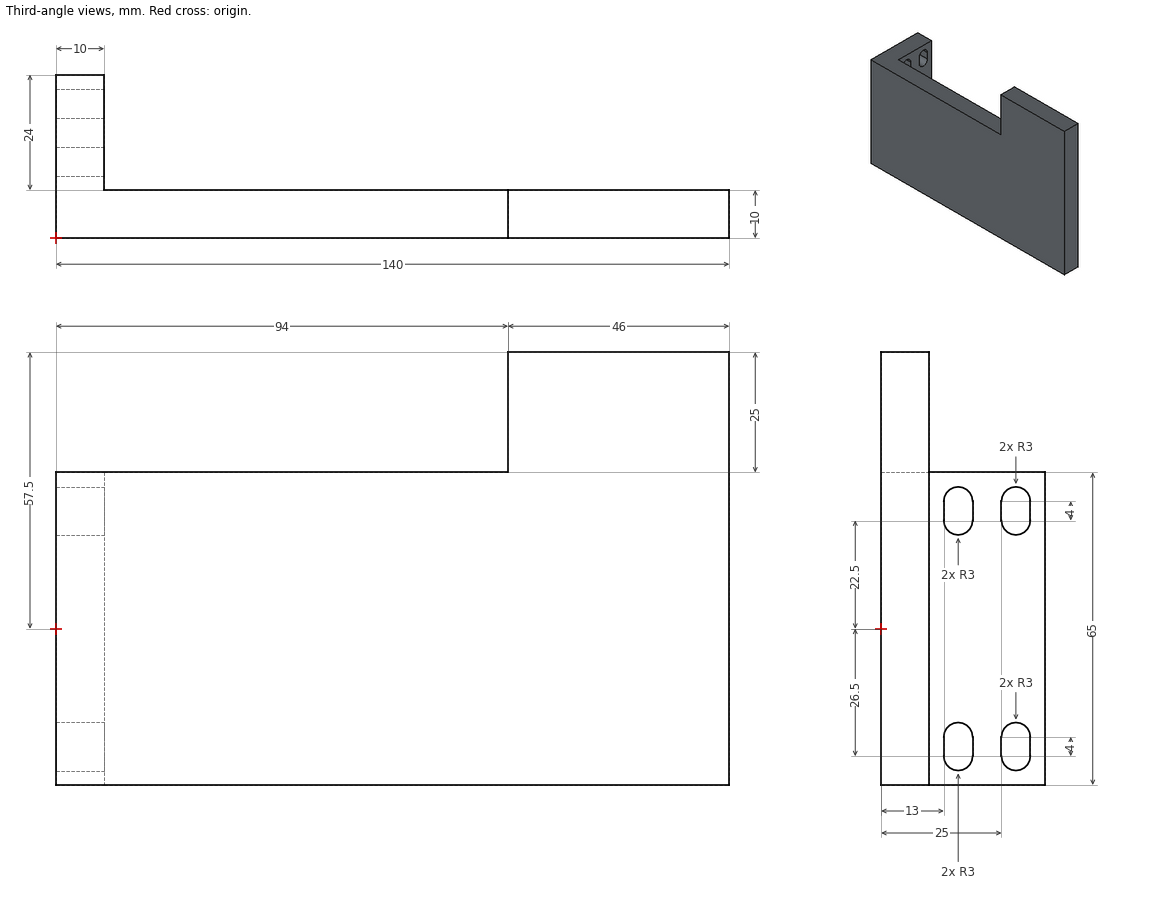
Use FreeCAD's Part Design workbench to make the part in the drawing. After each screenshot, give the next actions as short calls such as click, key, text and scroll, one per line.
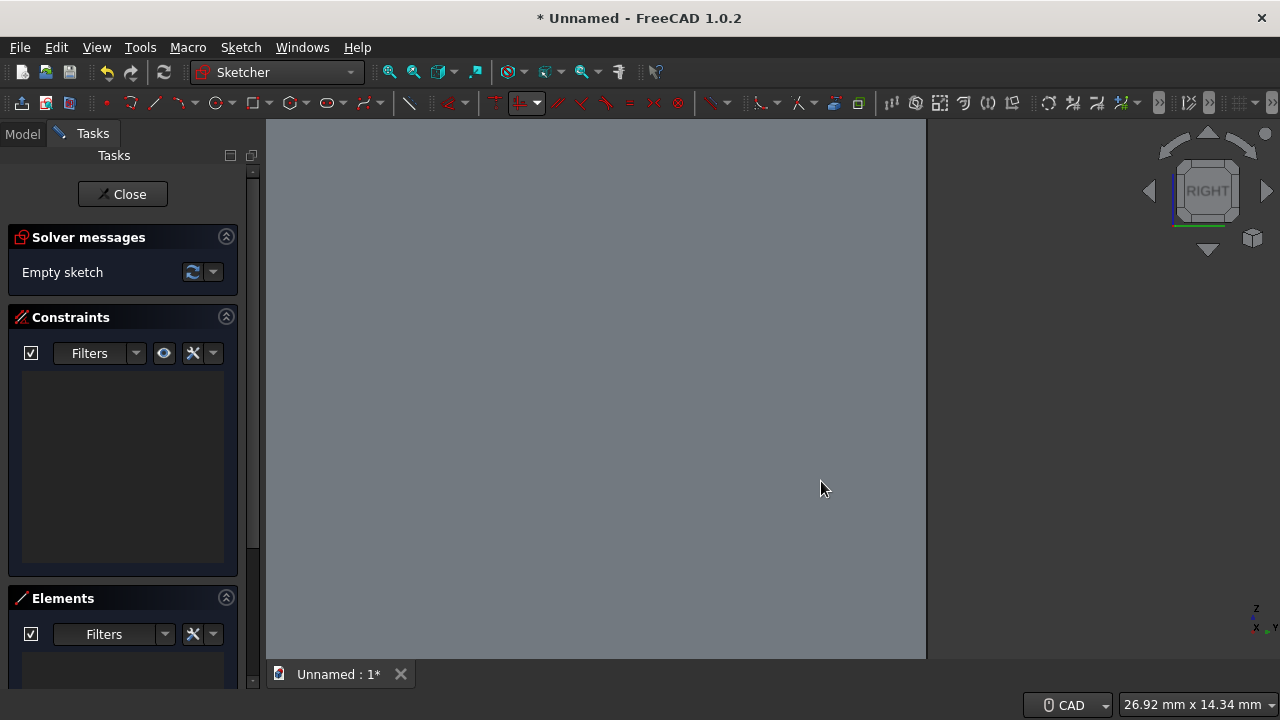
key(g)
key(s)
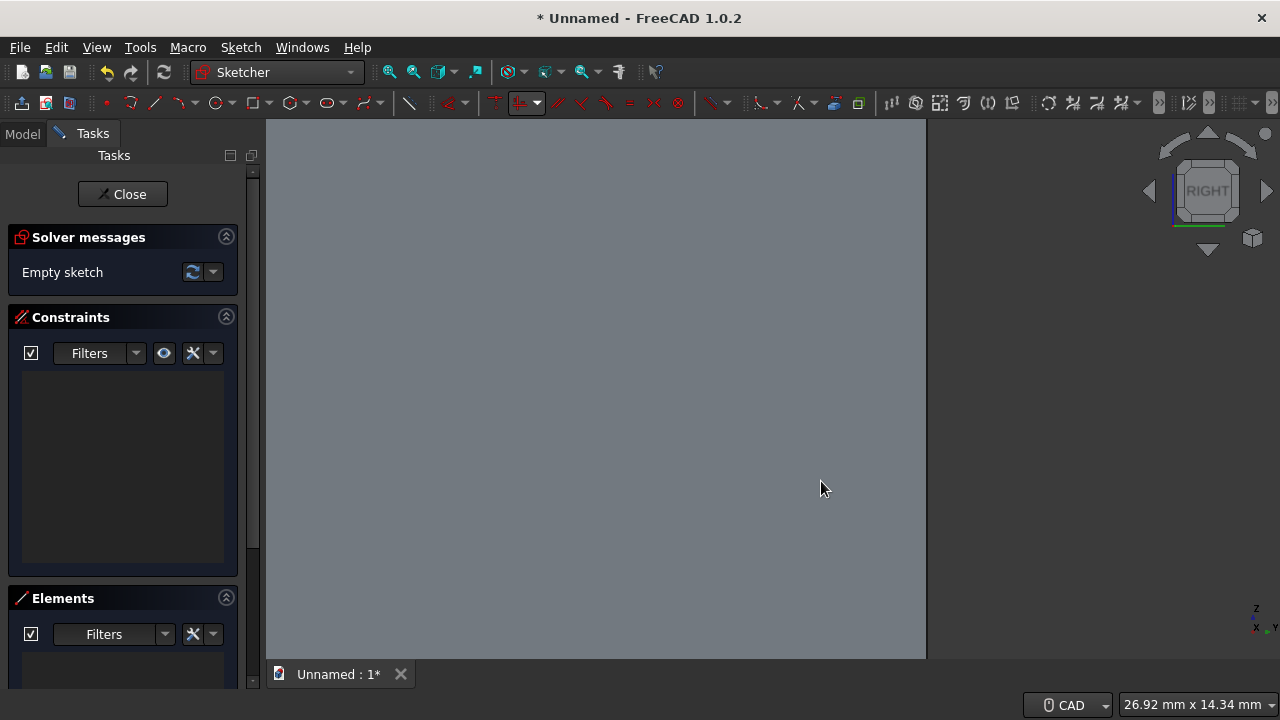
click(701, 458)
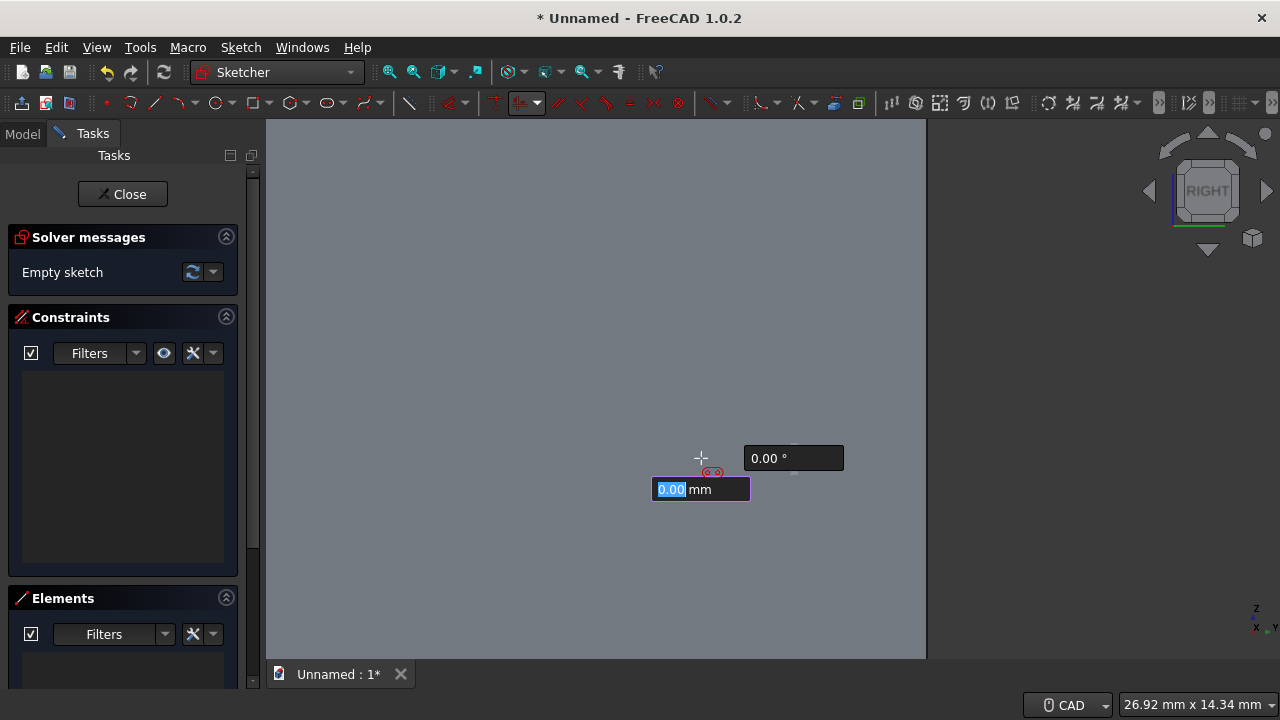
click(701, 308)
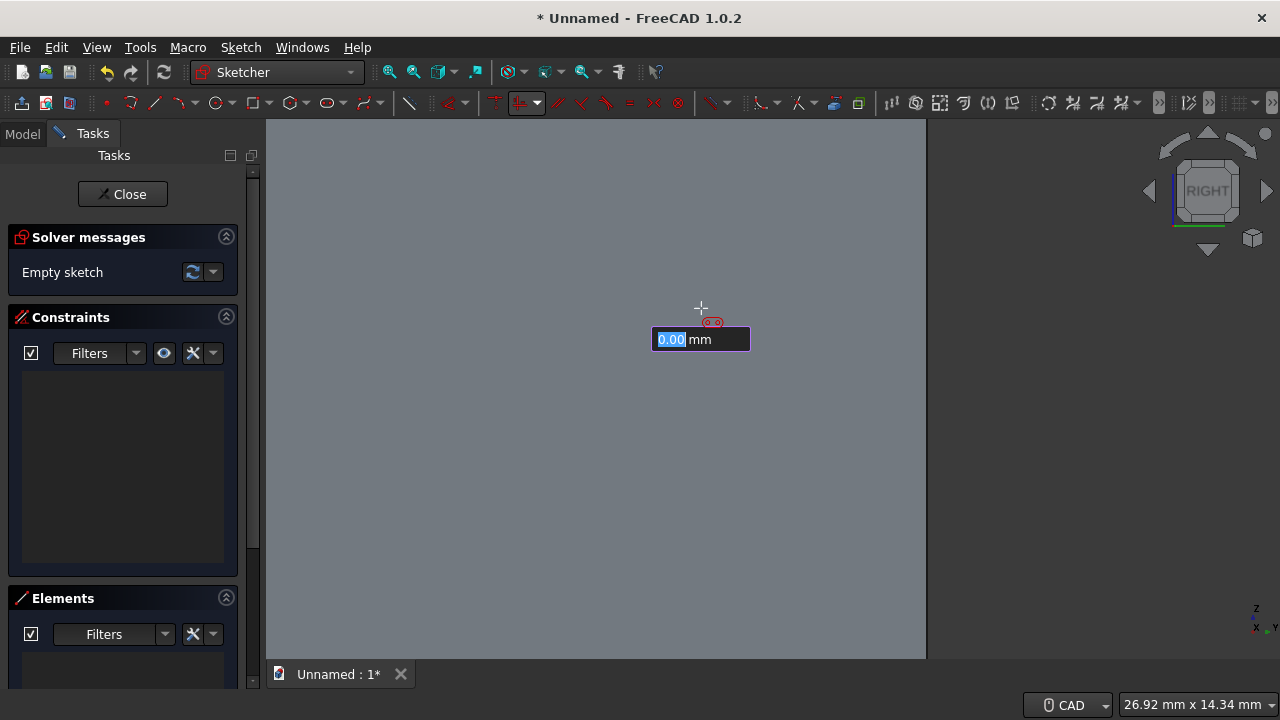
click(814, 383)
key(Escape)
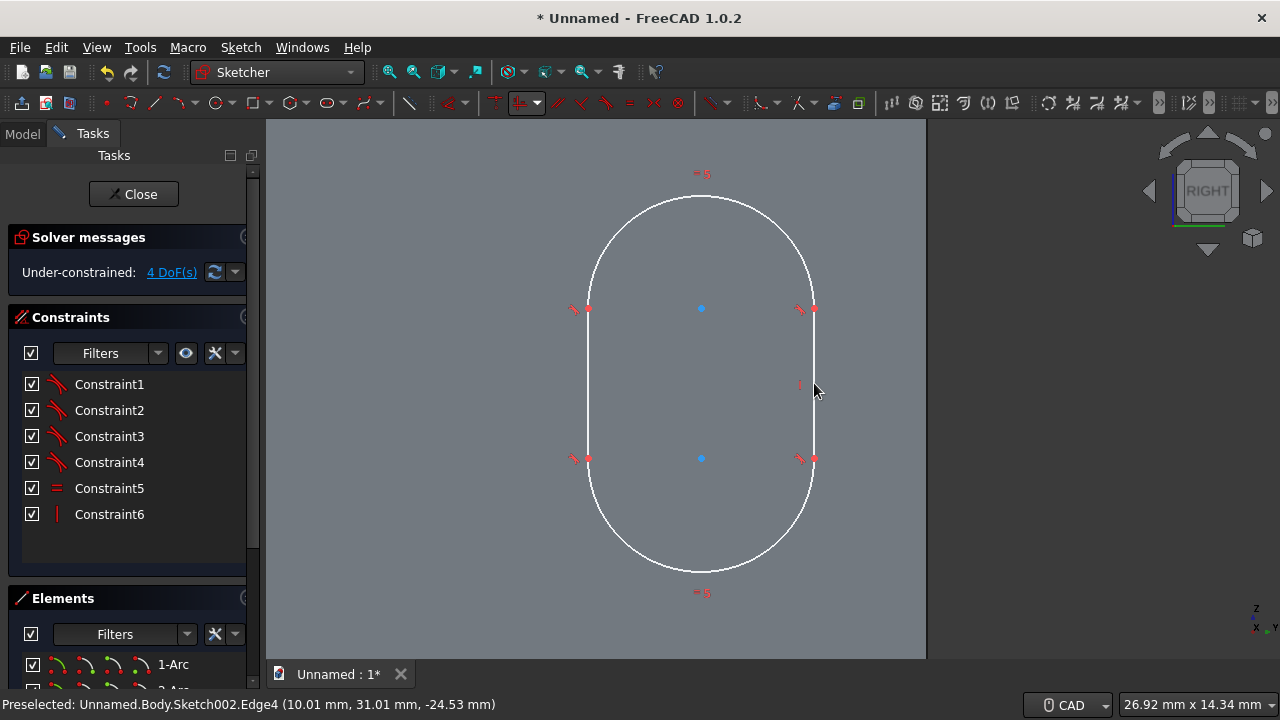
click(448, 104)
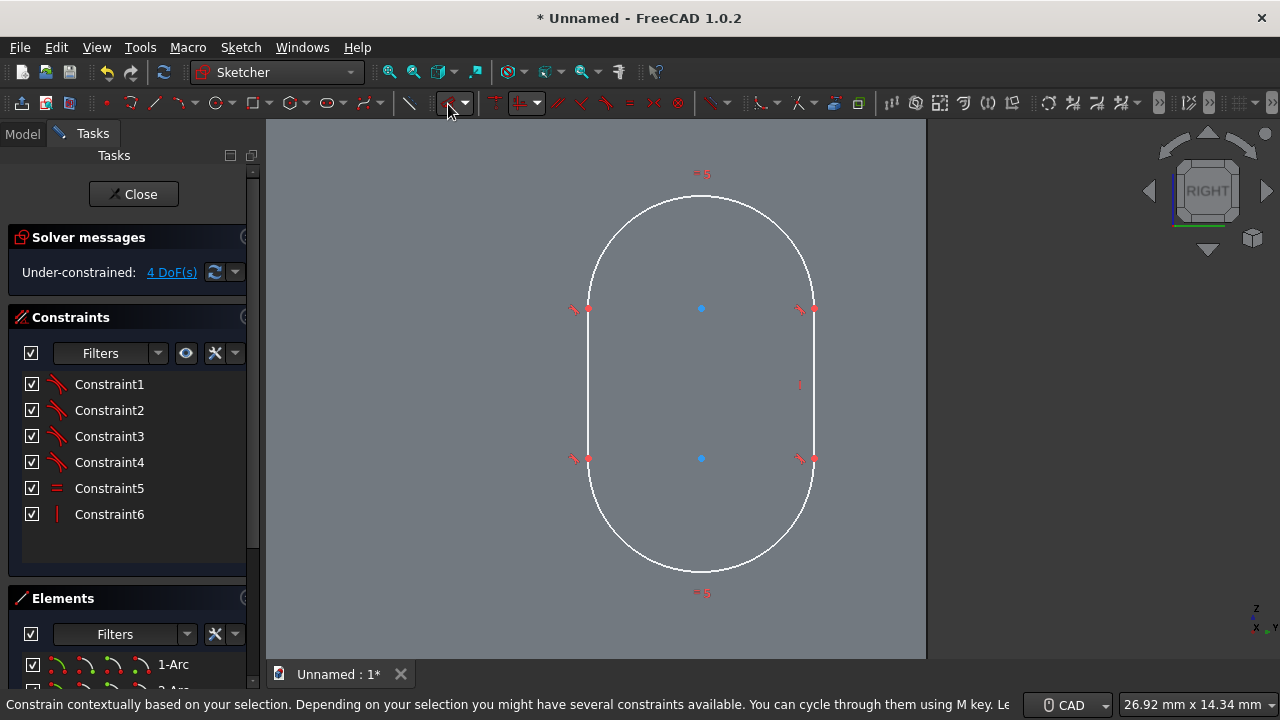
click(635, 550)
click(616, 576)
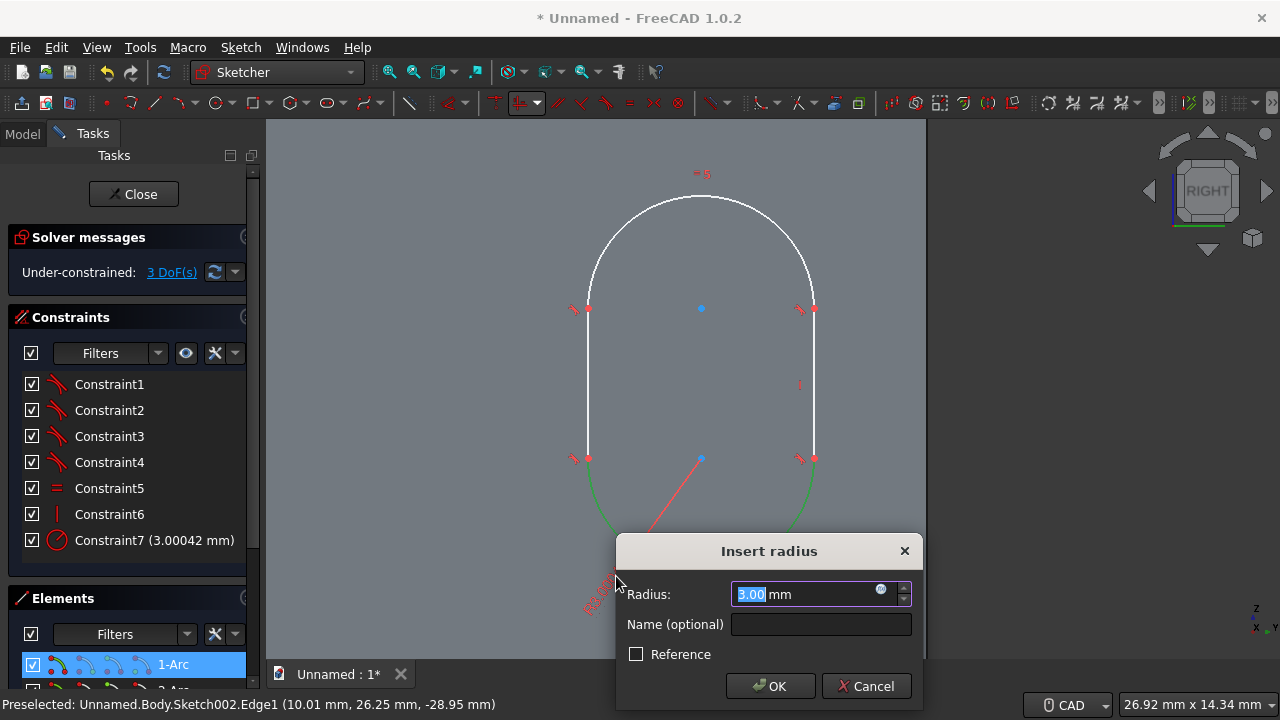
text(3)
key(Return)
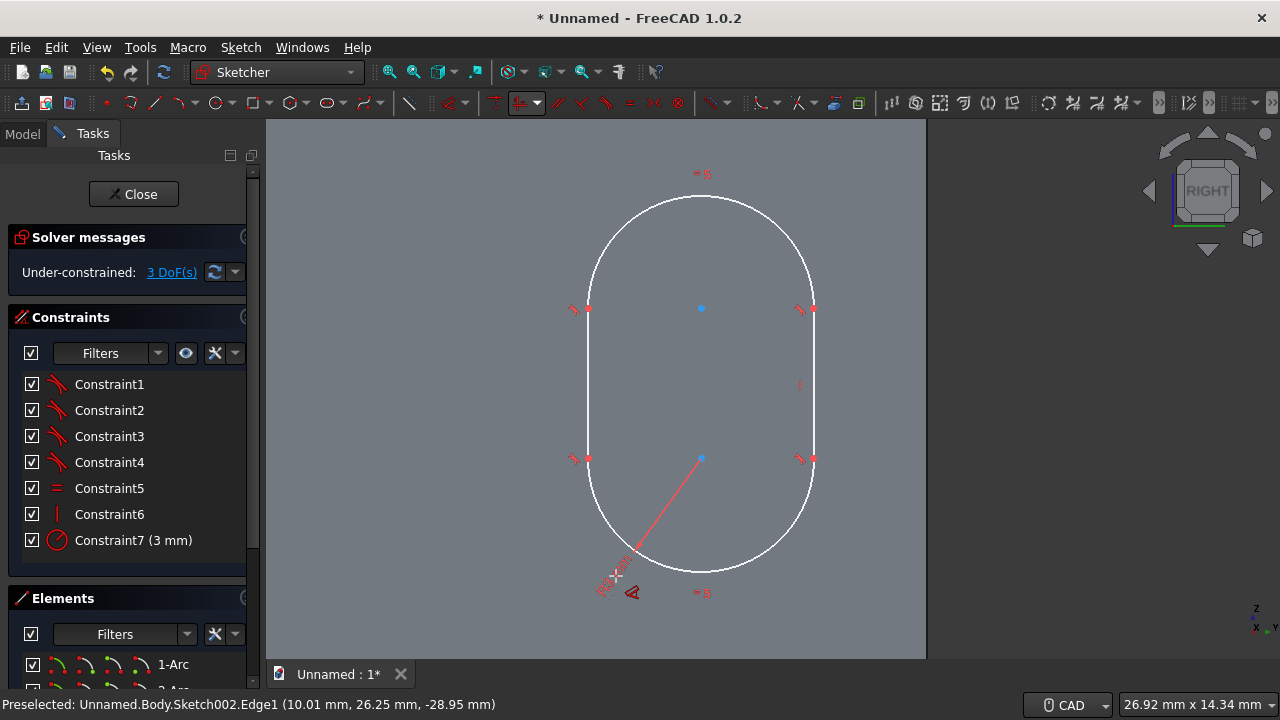
click(588, 414)
click(554, 384)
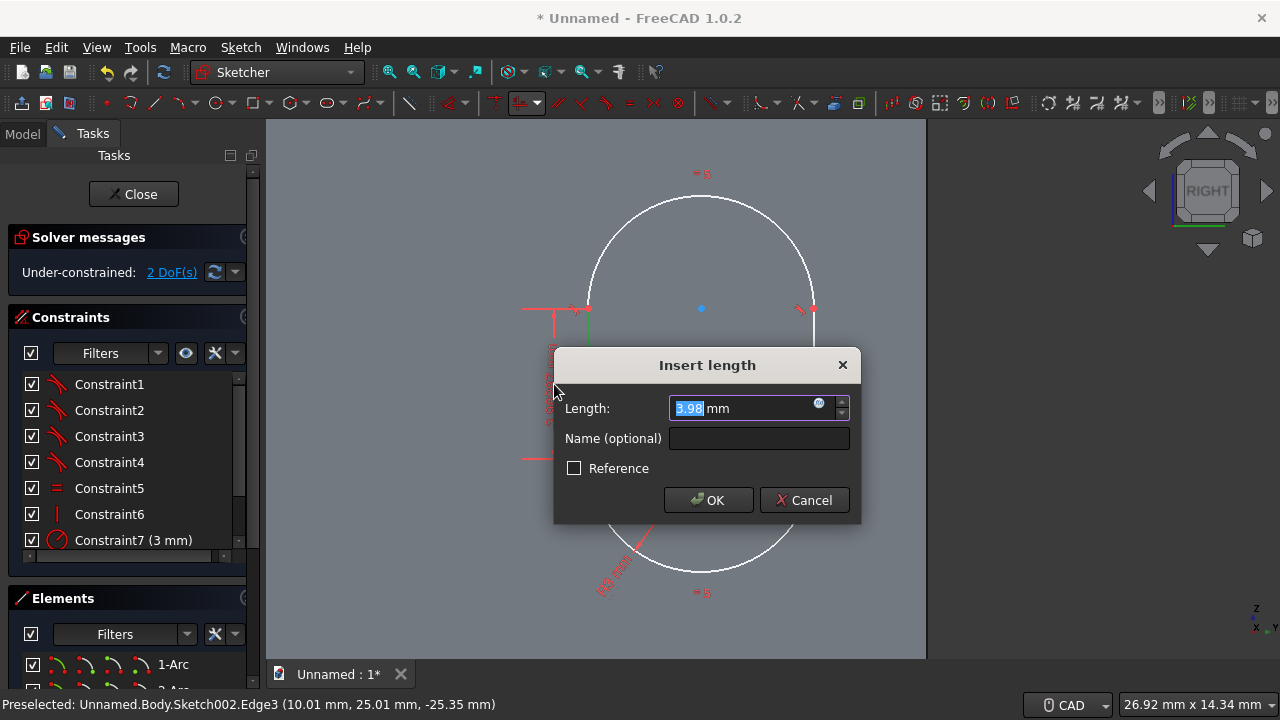
text(4)
key(Return)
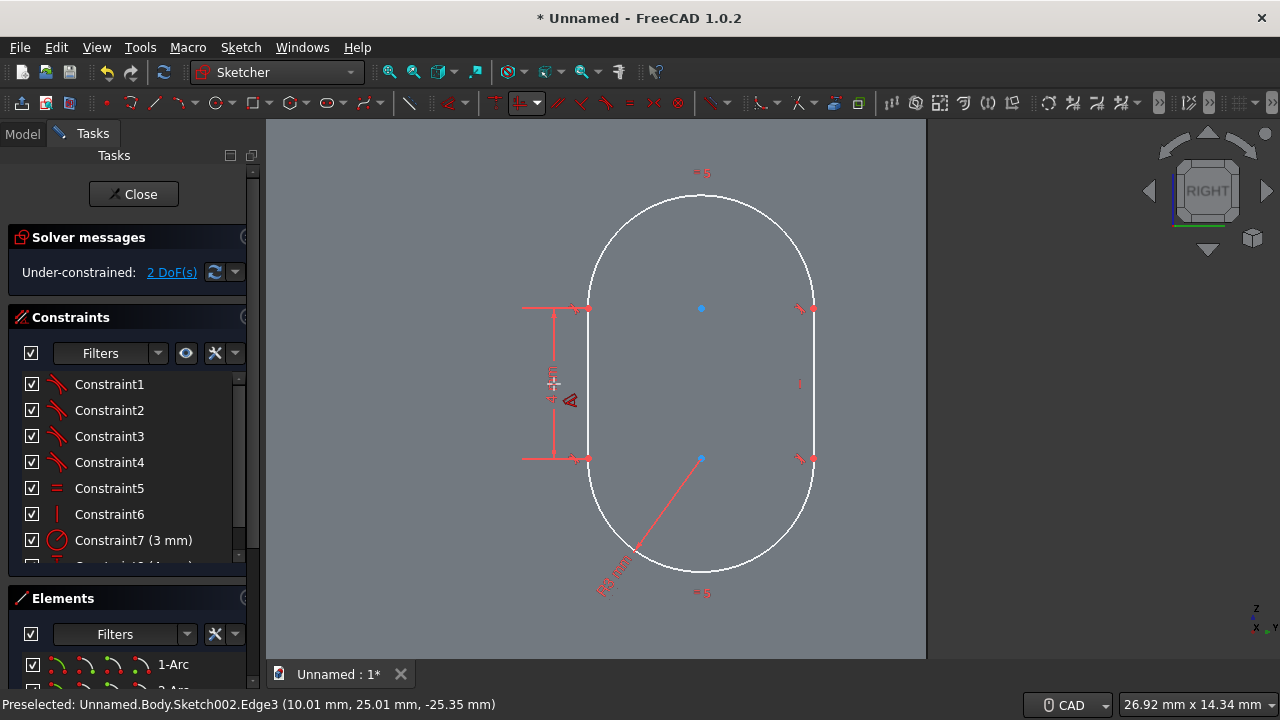
click(588, 459)
click(441, 493)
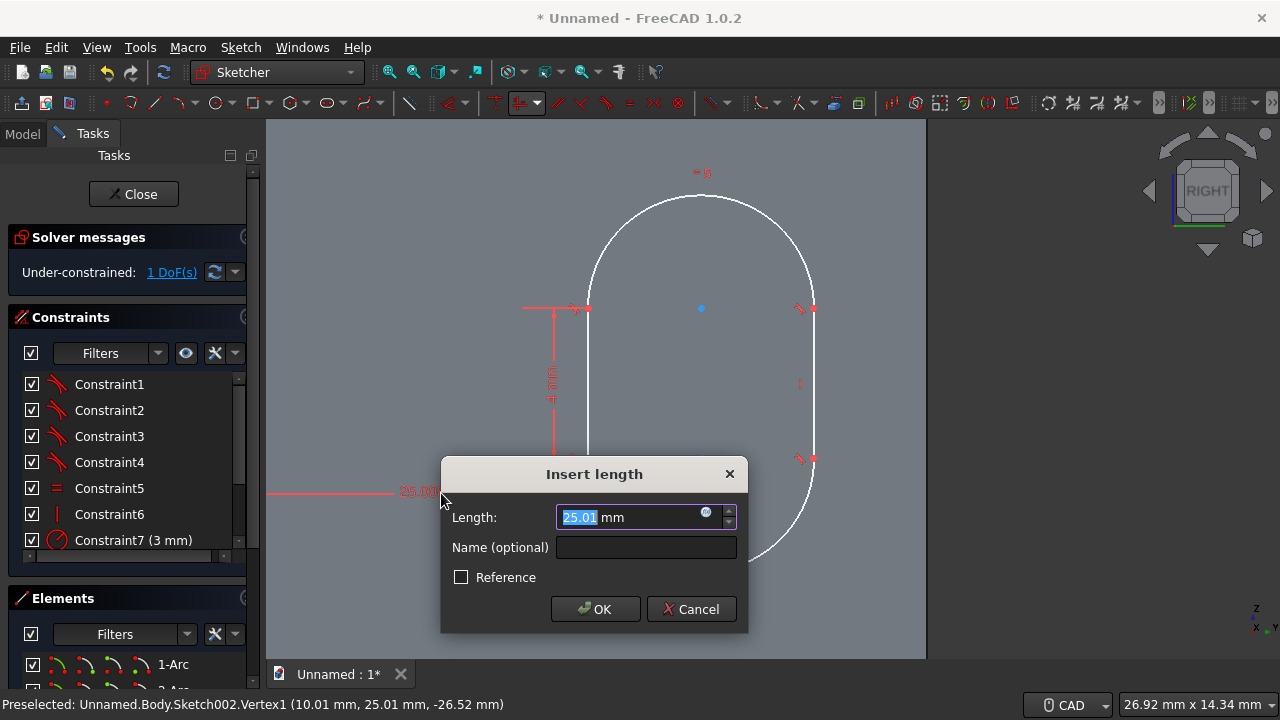
text(25)
key(Return)